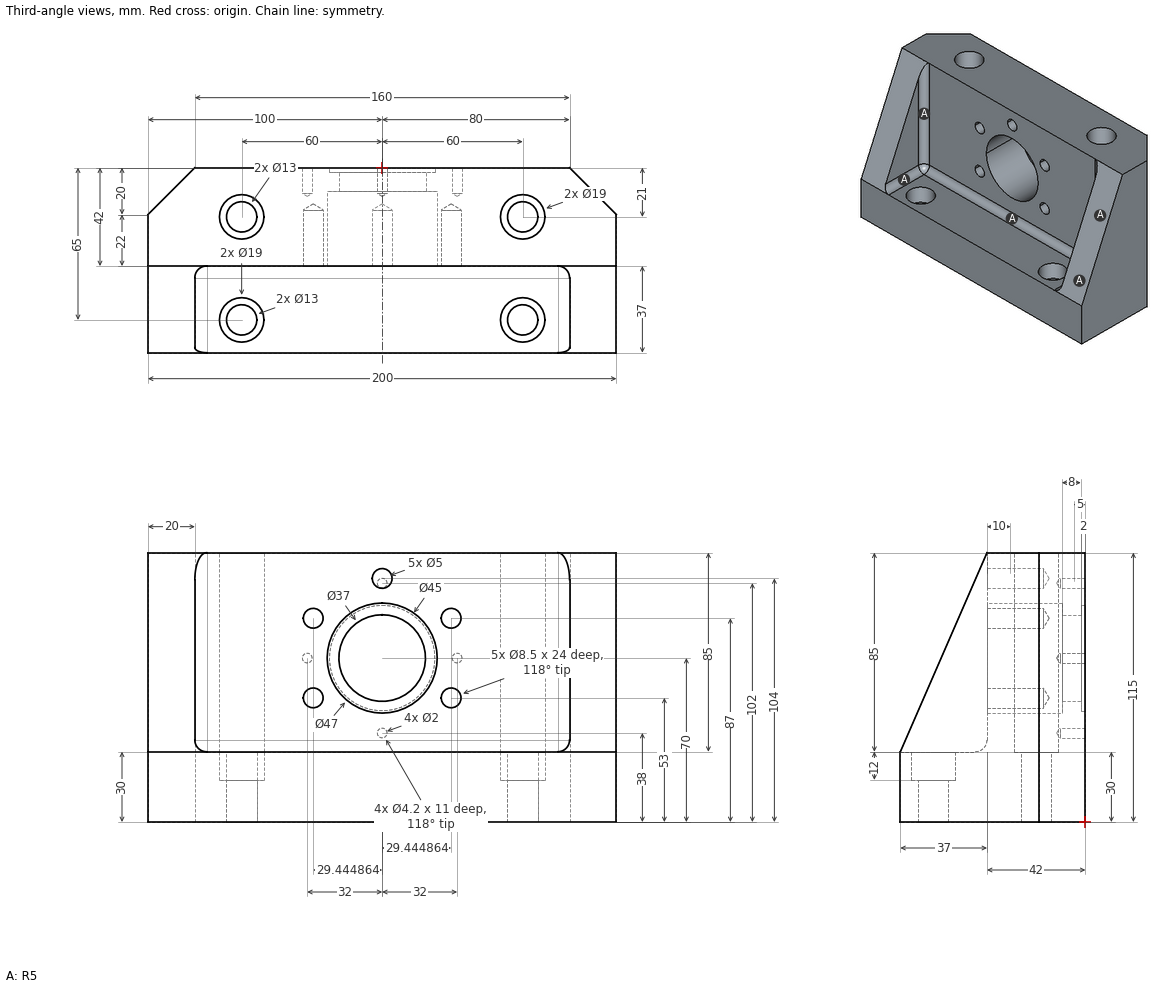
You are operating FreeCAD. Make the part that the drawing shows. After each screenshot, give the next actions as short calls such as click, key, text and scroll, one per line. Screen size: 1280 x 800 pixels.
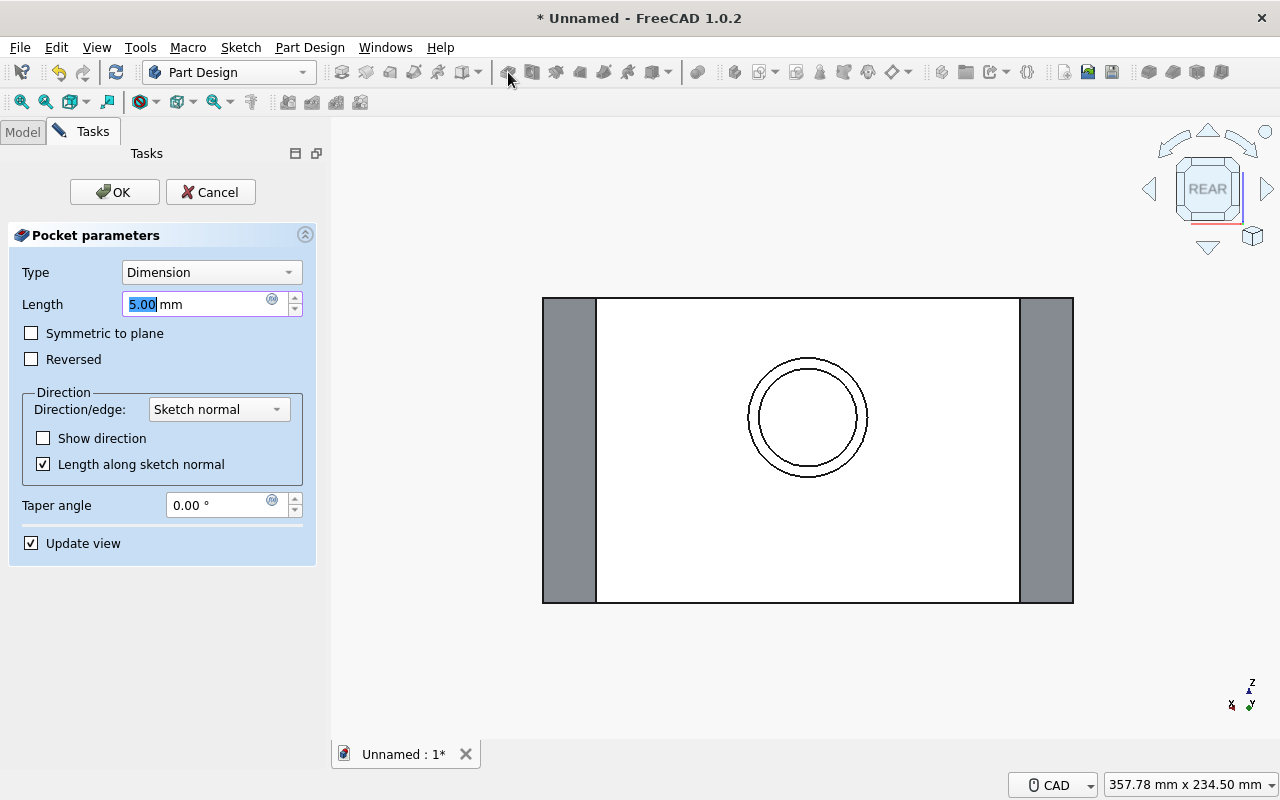
click(212, 272)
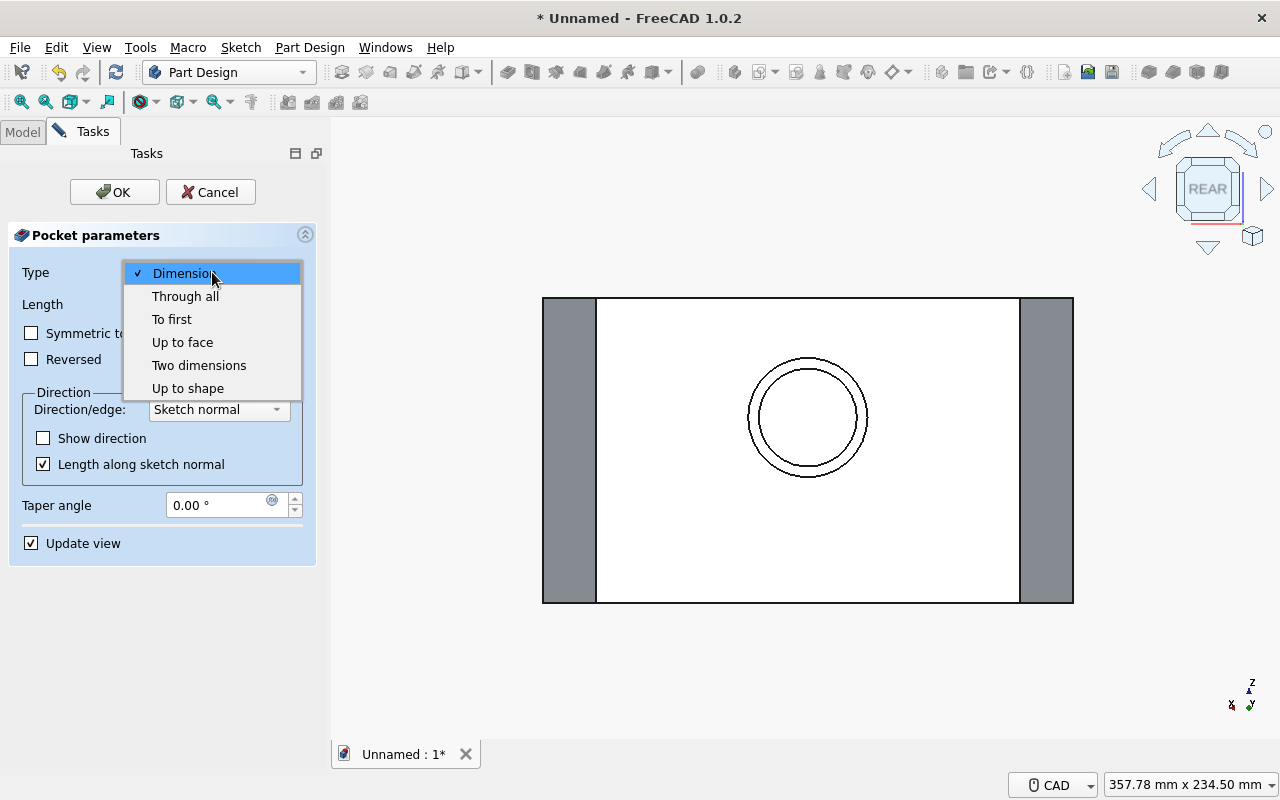
click(212, 320)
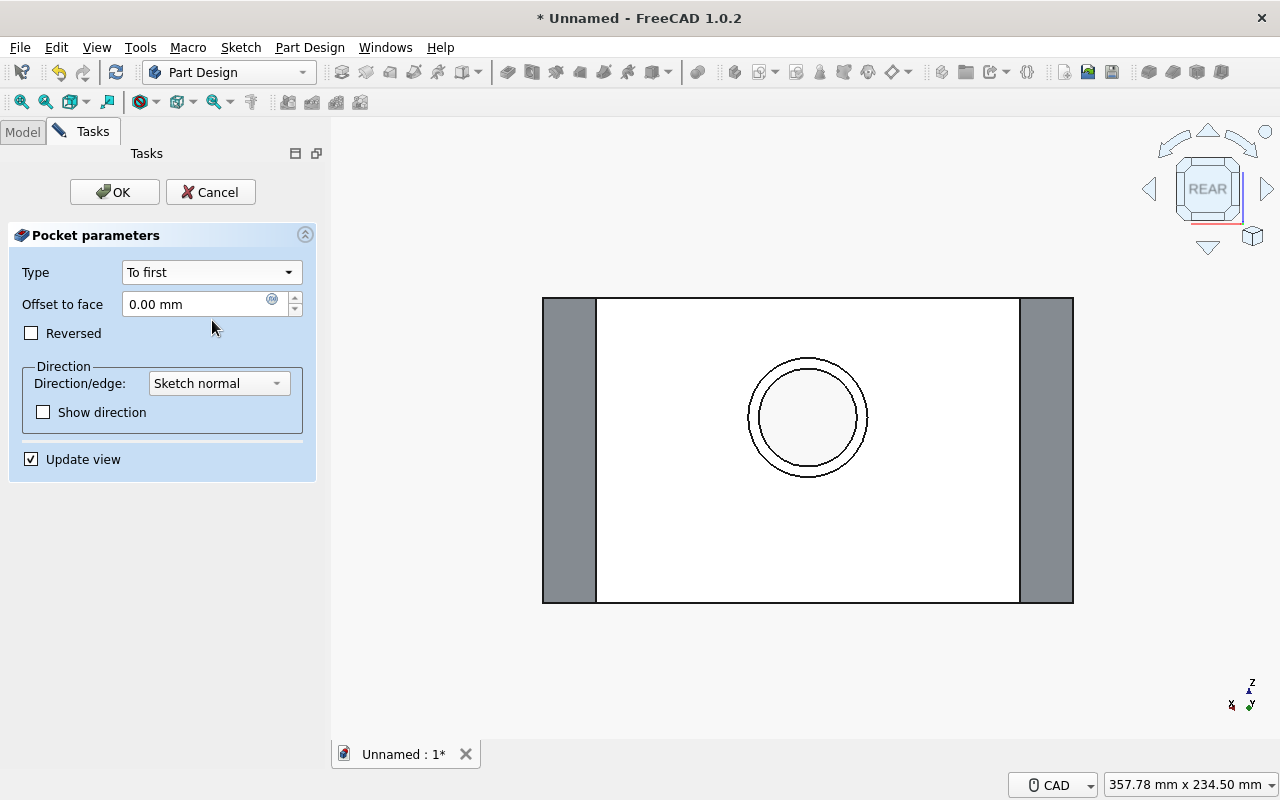
click(115, 192)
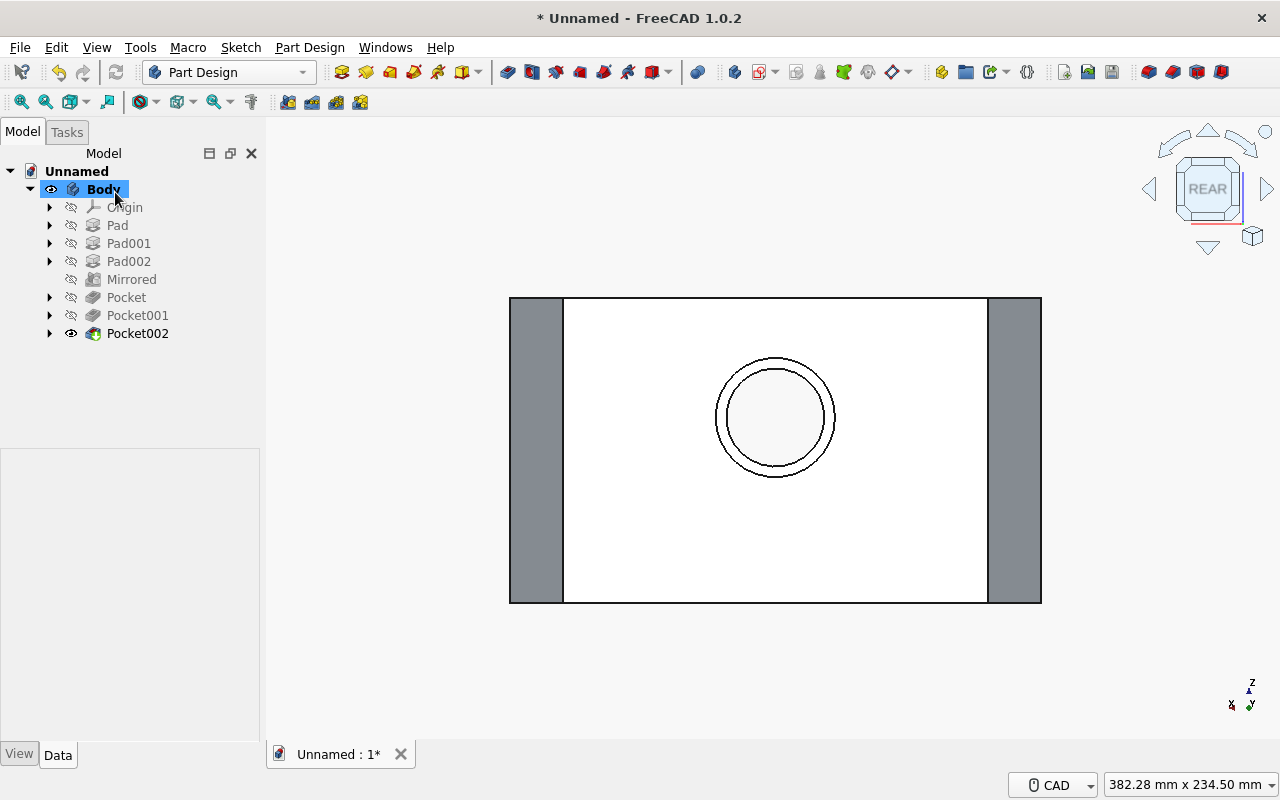
key(0)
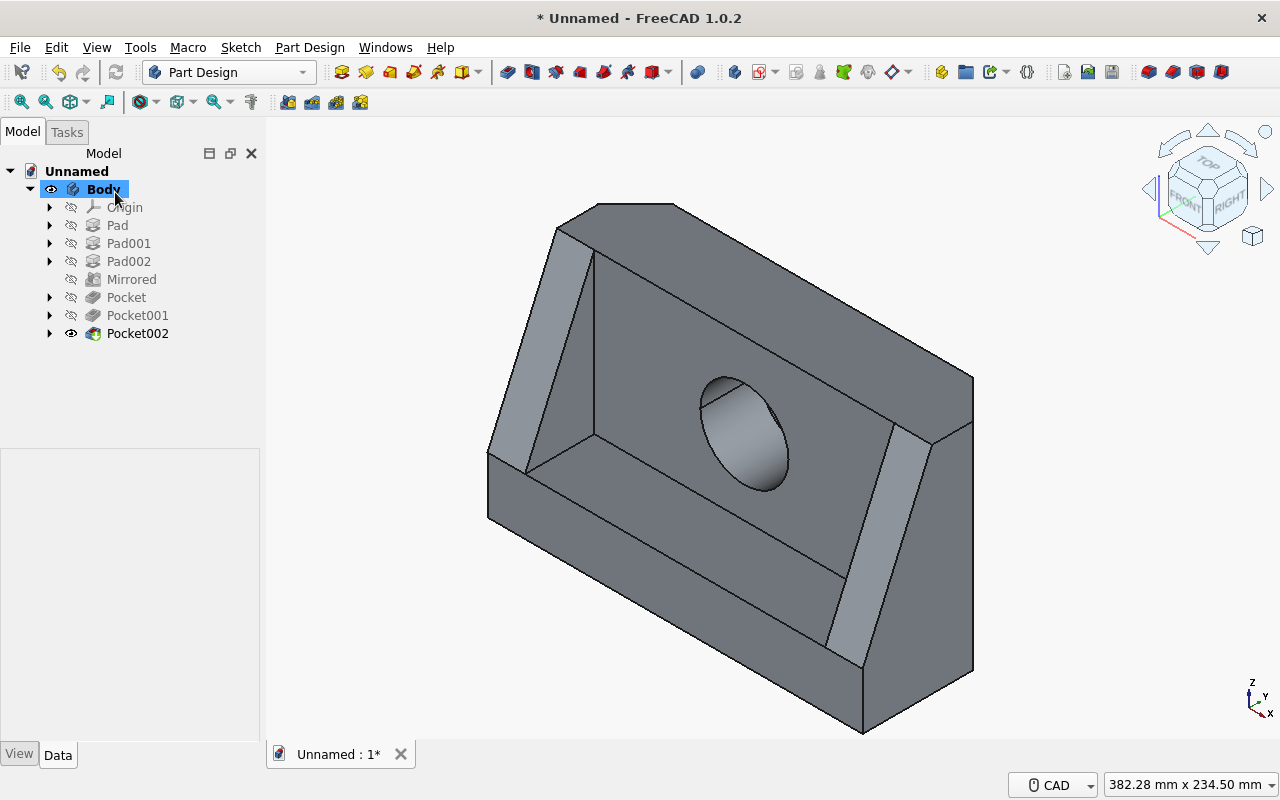
click(891, 375)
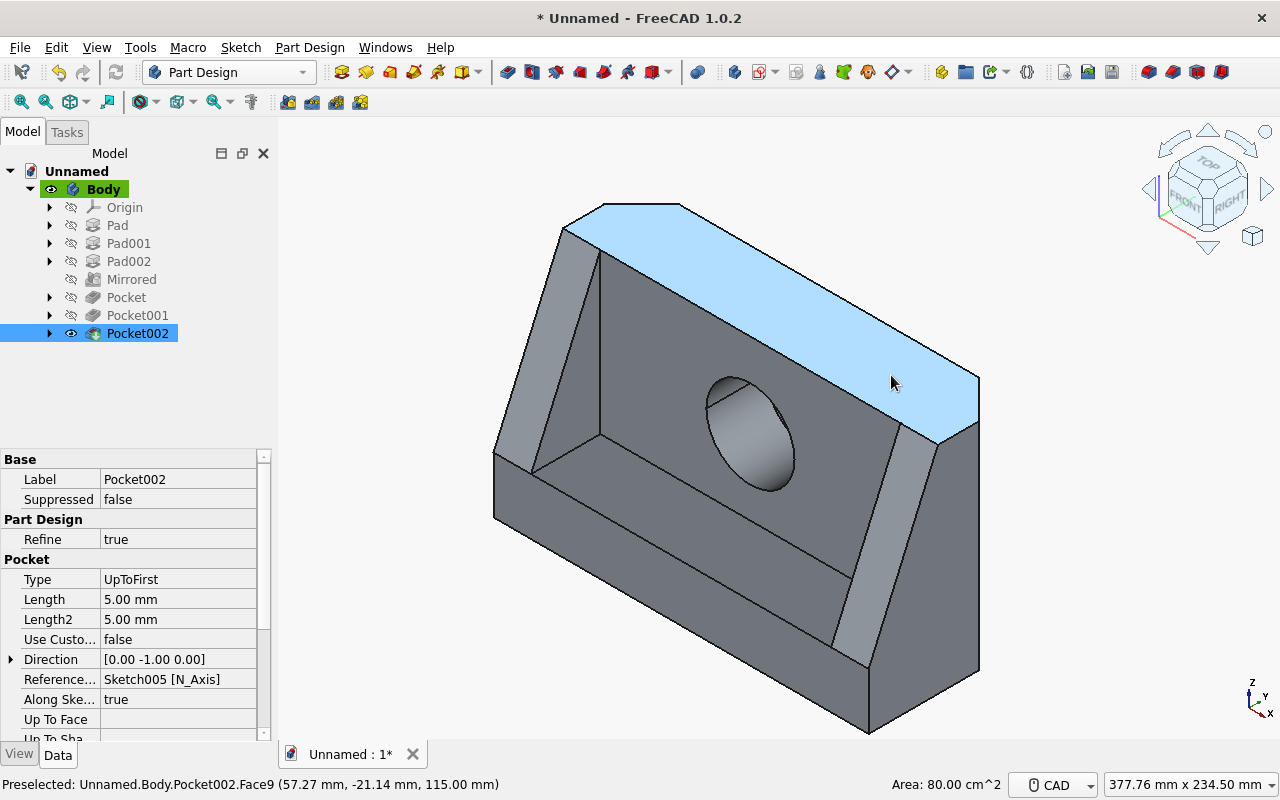
click(760, 72)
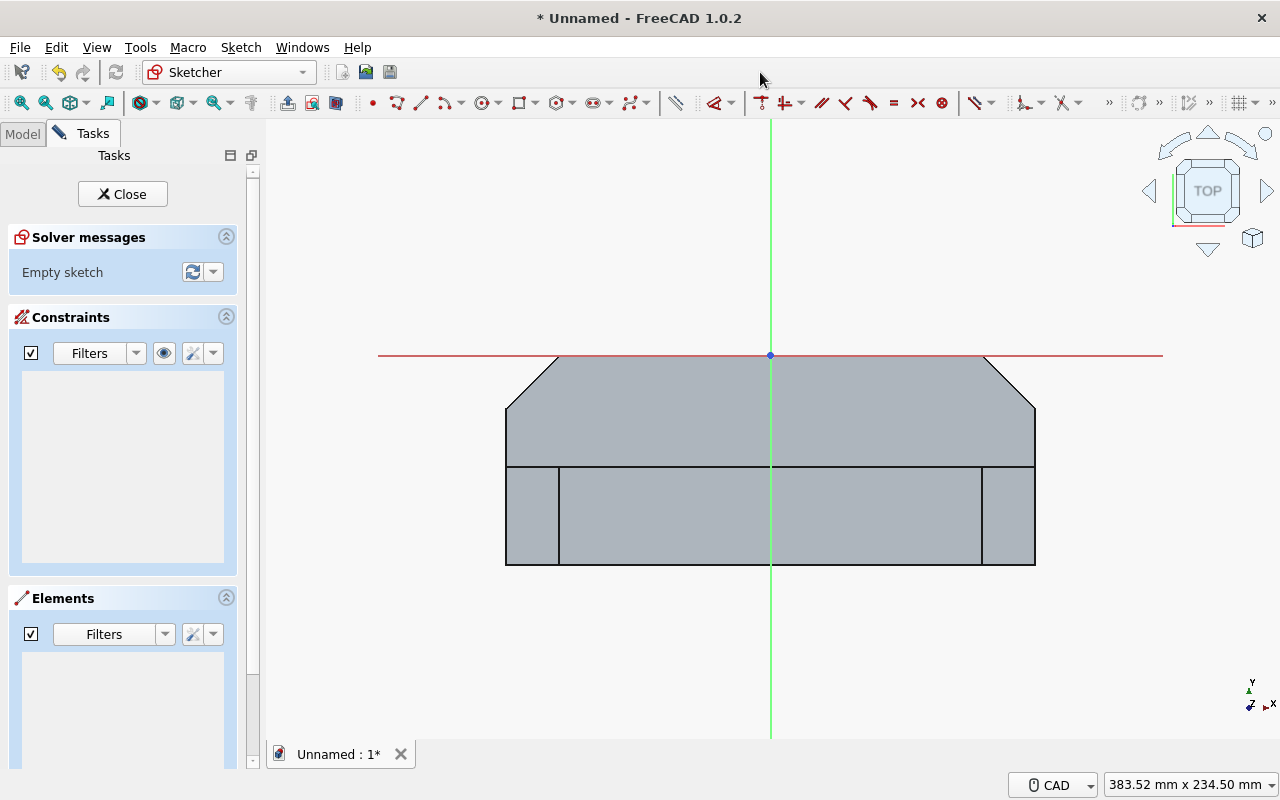
scroll(905, 329, up, 2)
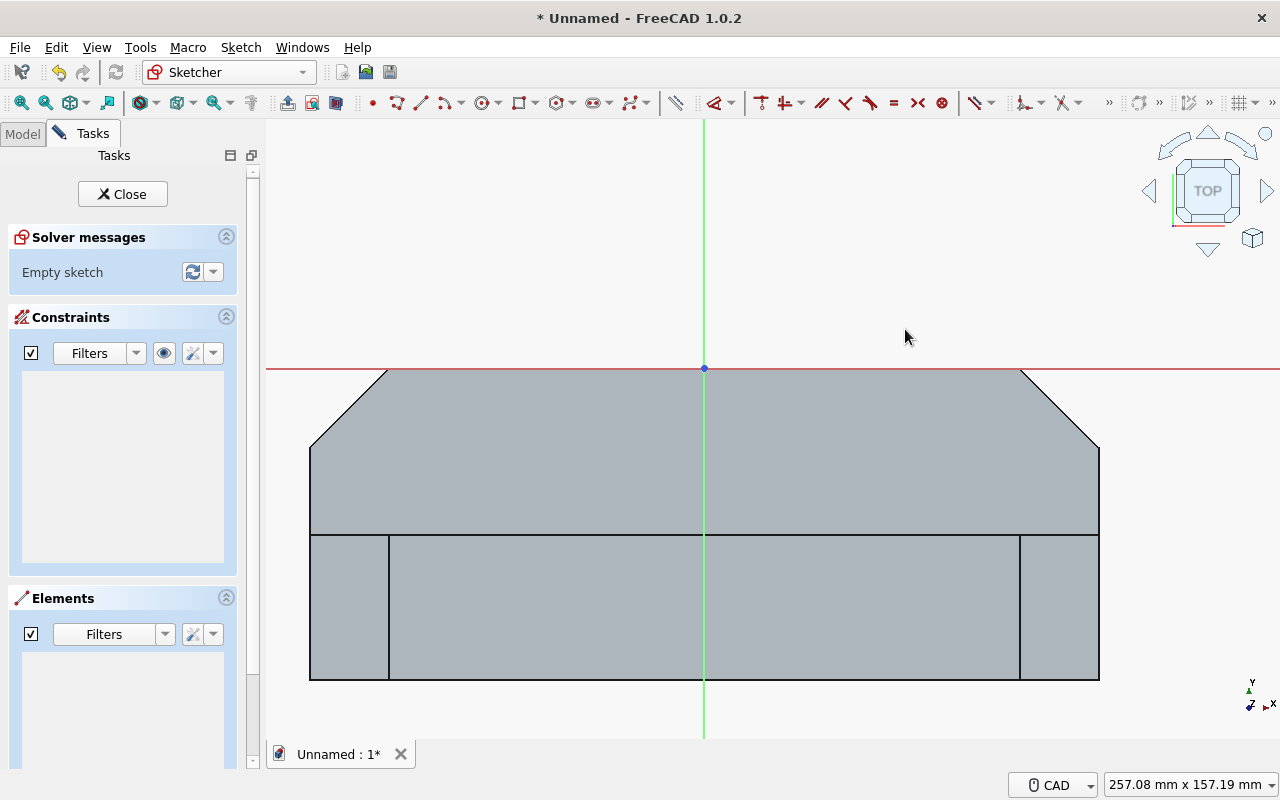
click(482, 104)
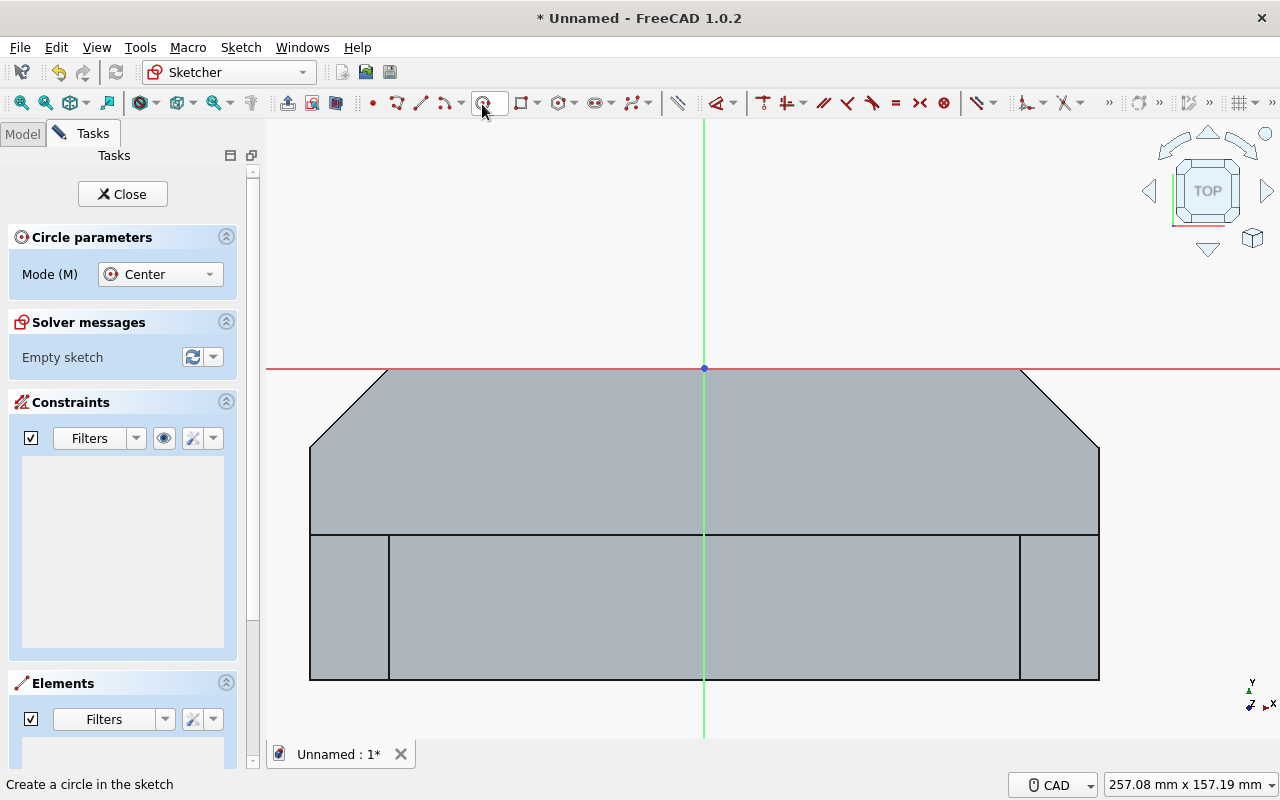
click(941, 452)
move(967, 425)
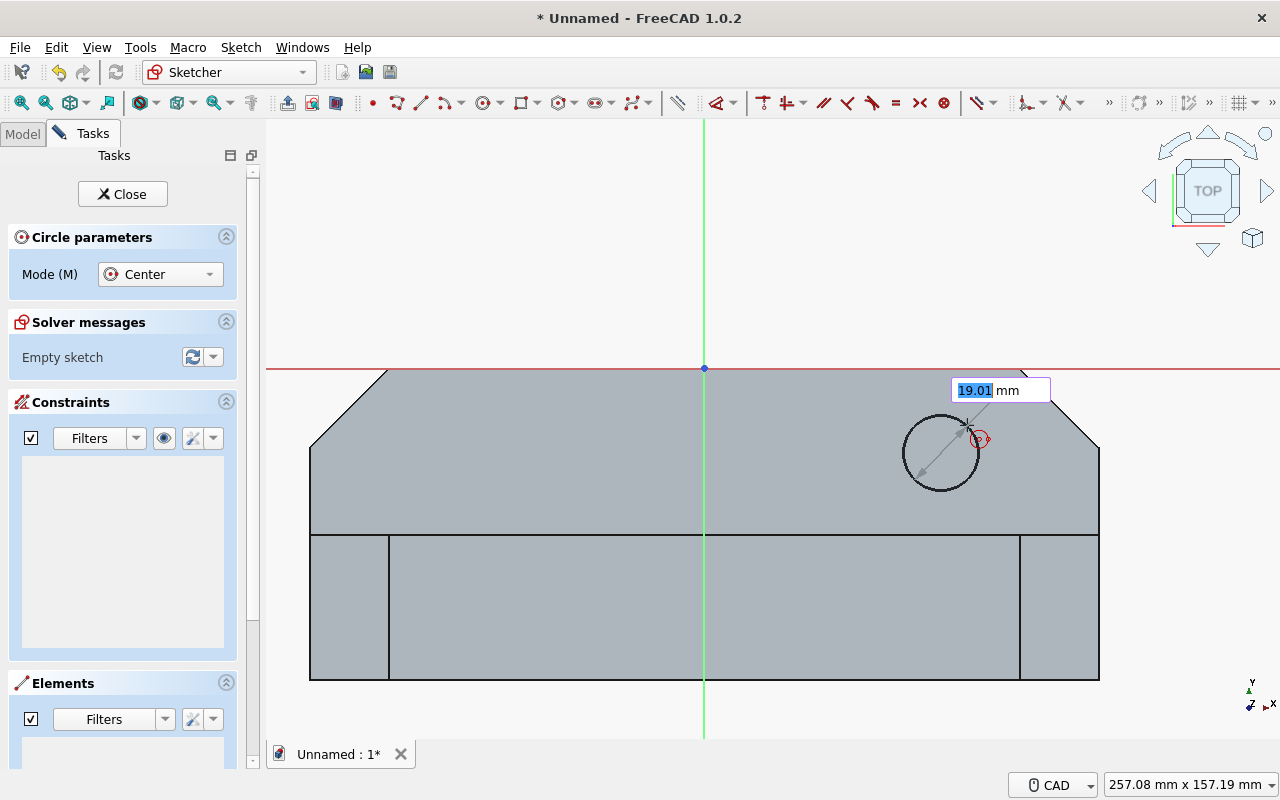
text(19)
key(Return)